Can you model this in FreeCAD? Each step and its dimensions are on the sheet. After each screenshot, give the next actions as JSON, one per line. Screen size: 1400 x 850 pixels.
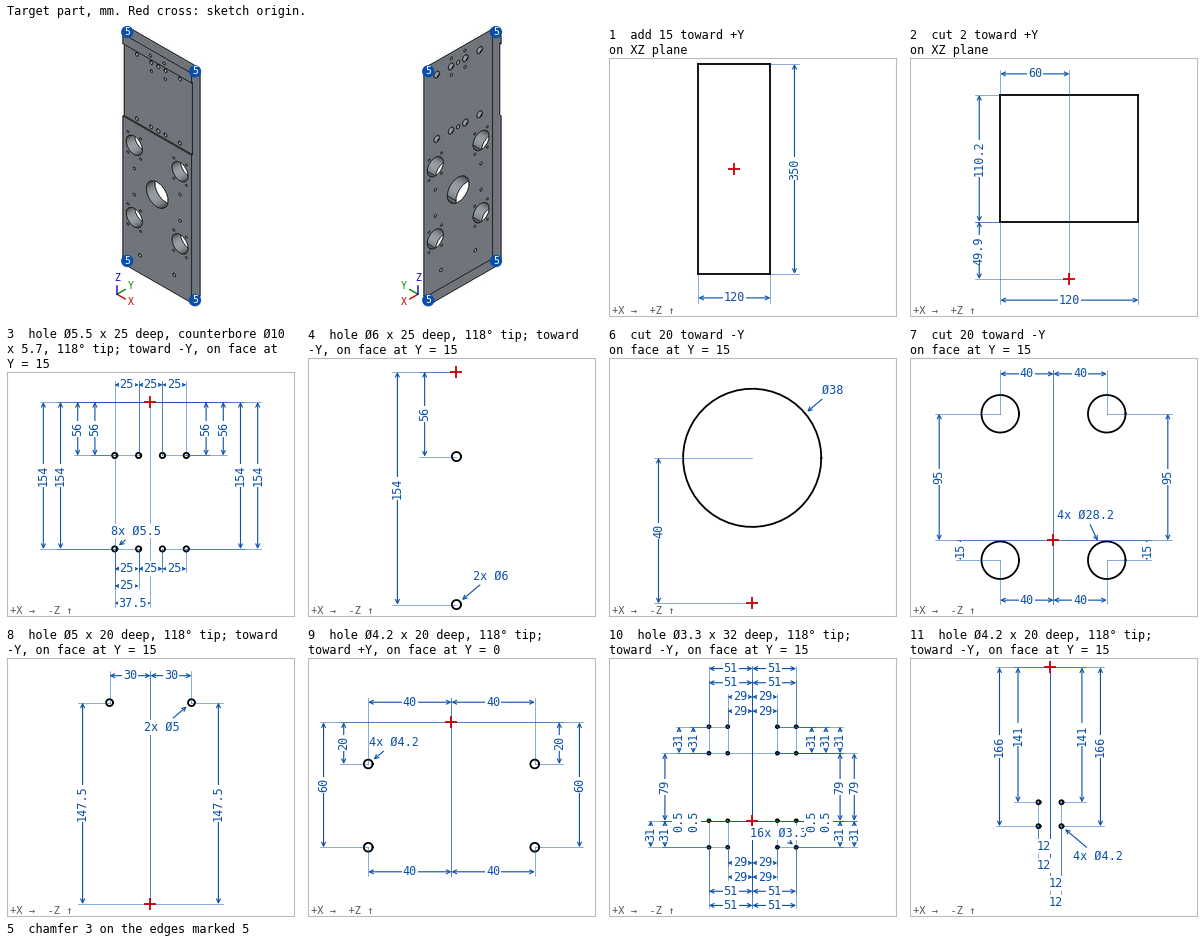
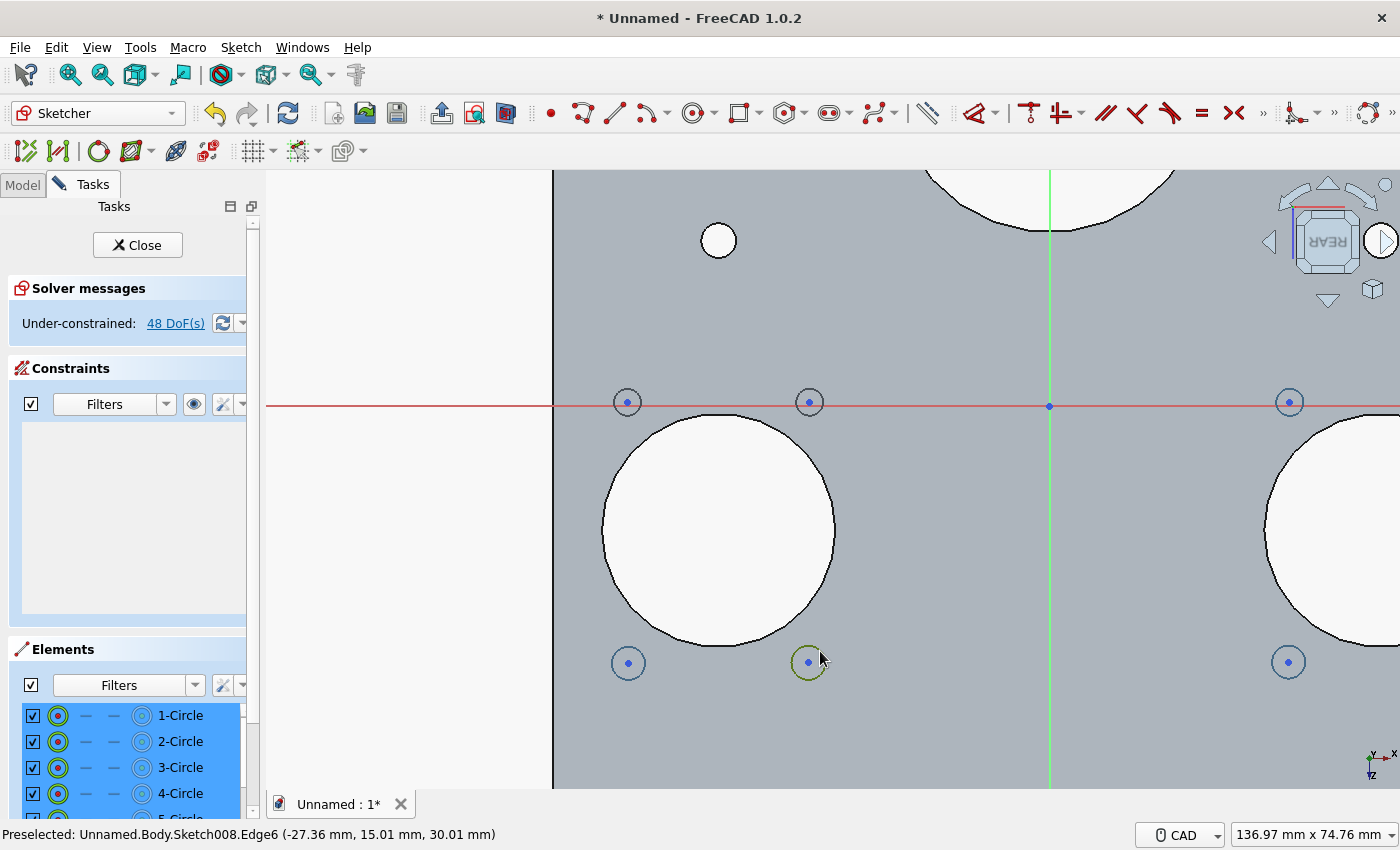
{"action": "left_click", "coordinate": [819, 393]}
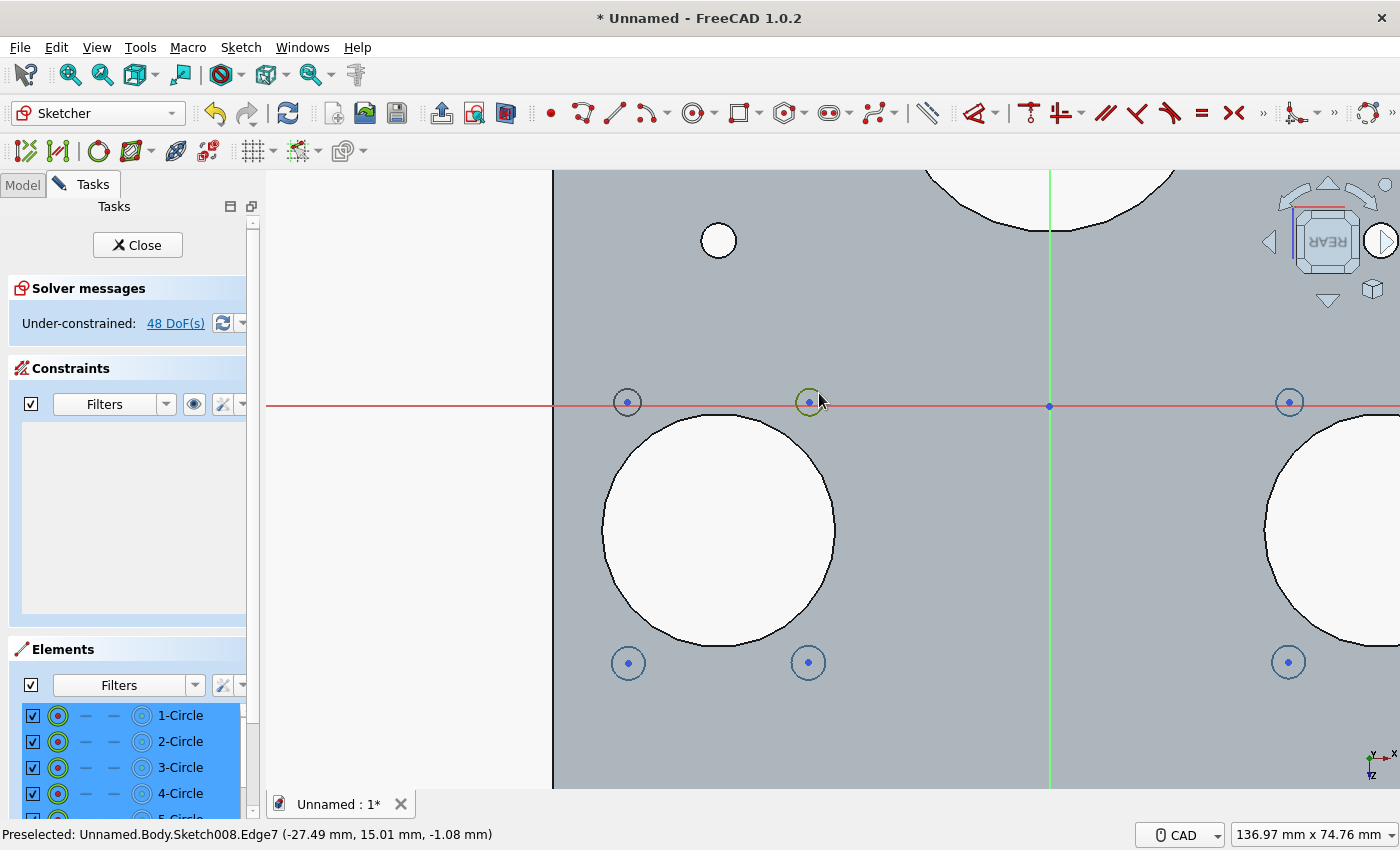
{"action": "left_click", "coordinate": [637, 393]}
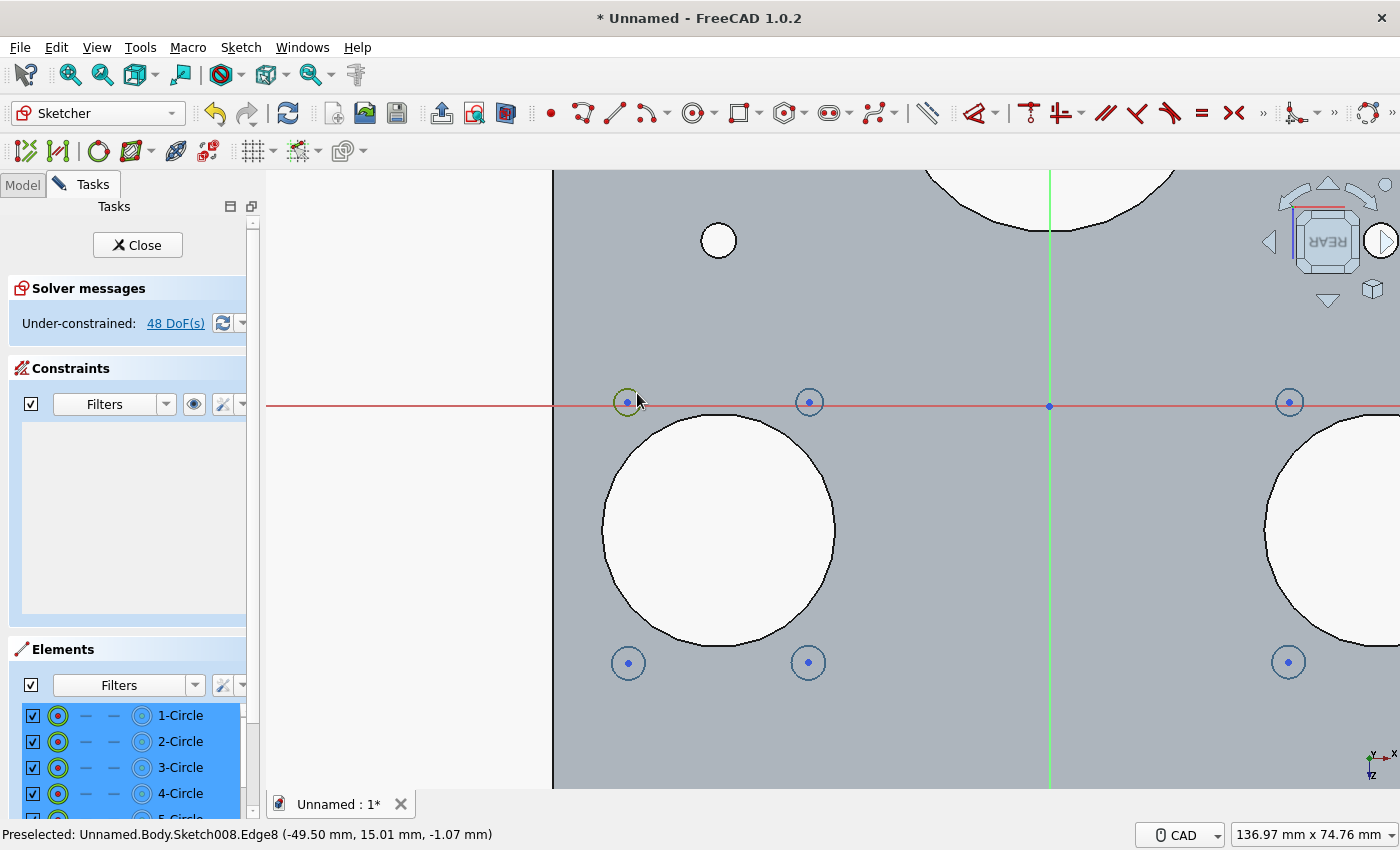
{"action": "scroll", "coordinate": [642, 654], "scroll_direction": "down", "scroll_amount": 6}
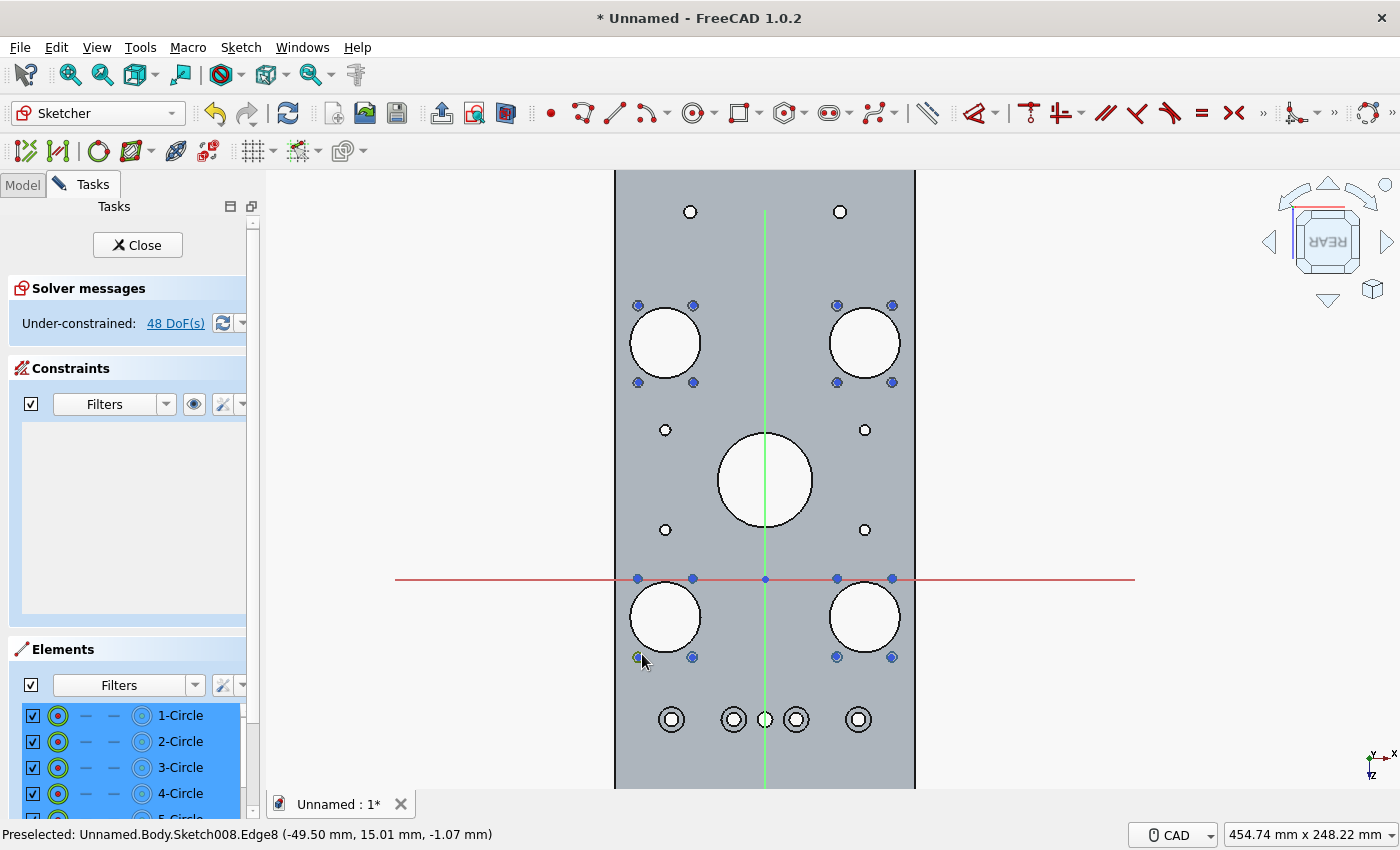
{"action": "scroll", "coordinate": [895, 379], "scroll_direction": "up", "scroll_amount": 6}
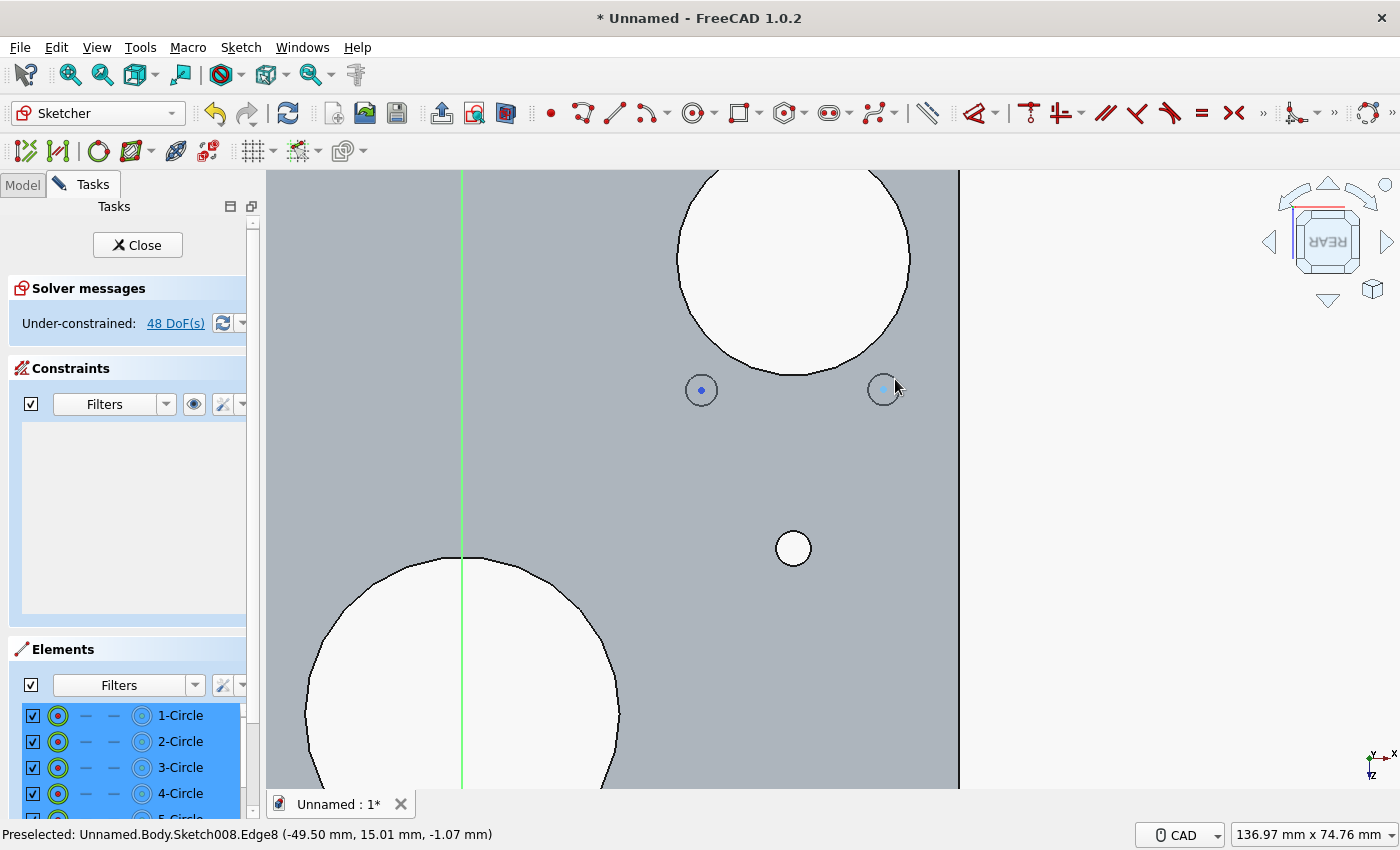
{"action": "left_click", "coordinate": [895, 379]}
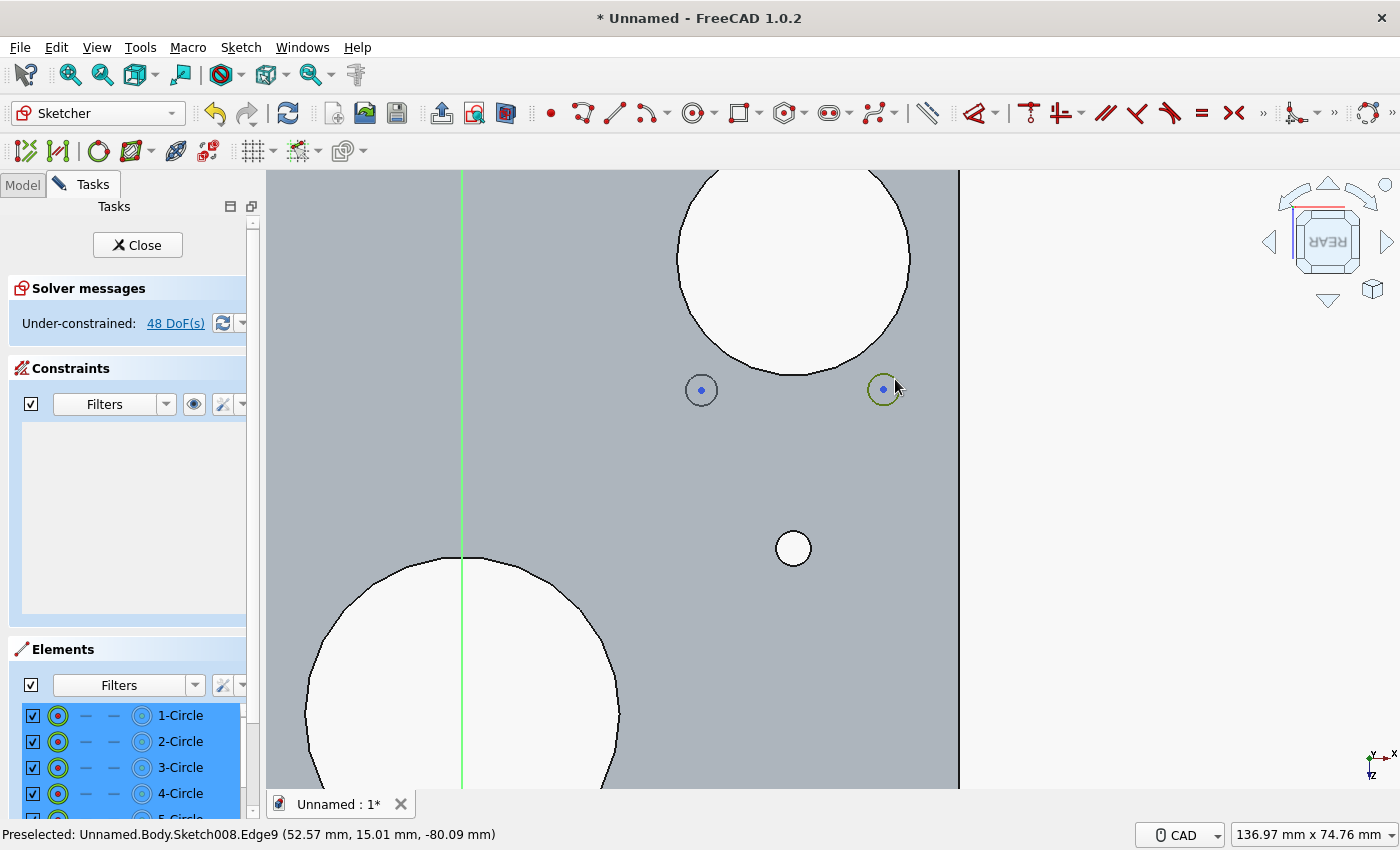
{"action": "left_click", "coordinate": [713, 379]}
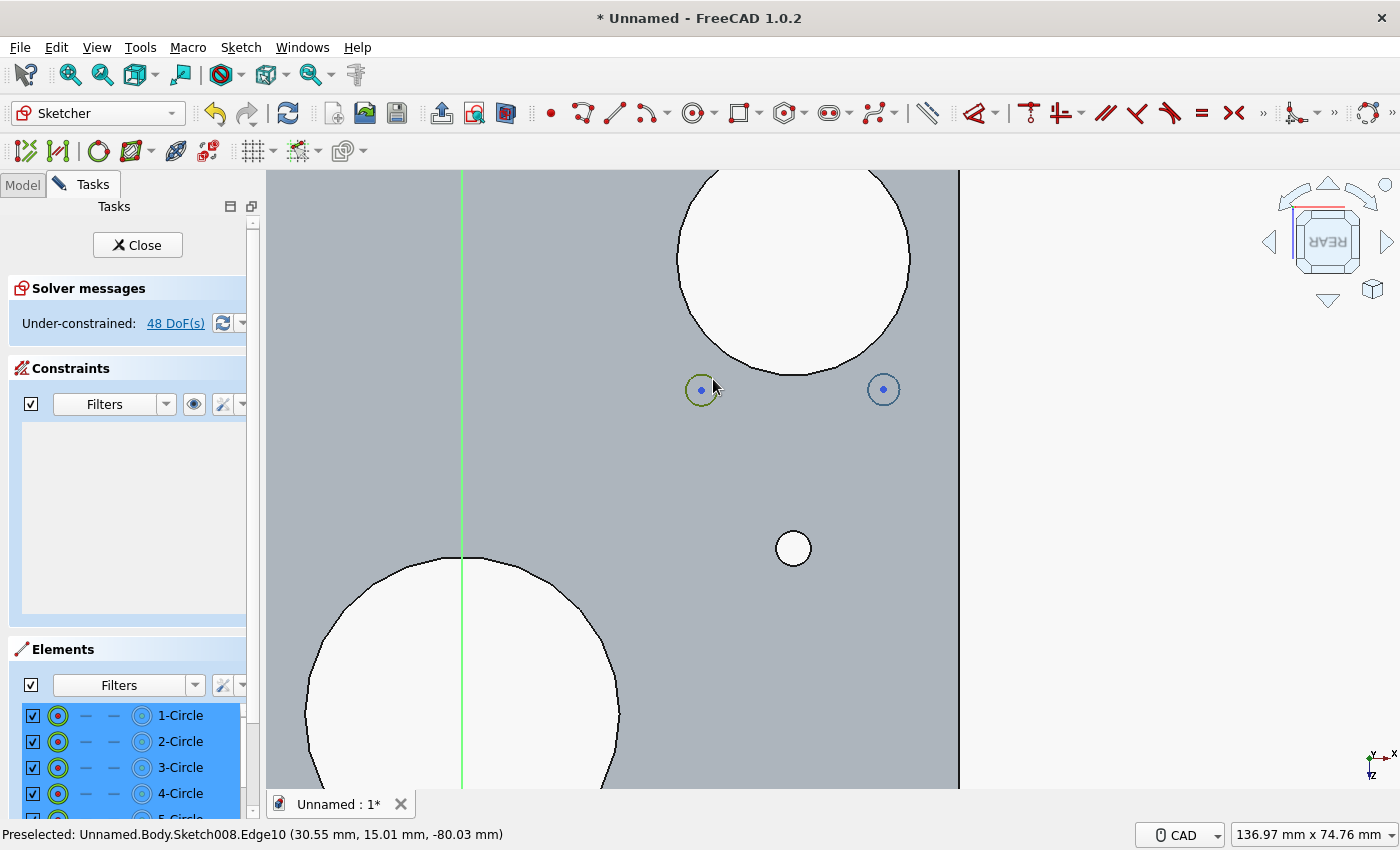
{"action": "scroll", "coordinate": [895, 378], "scroll_direction": "down", "scroll_amount": 6}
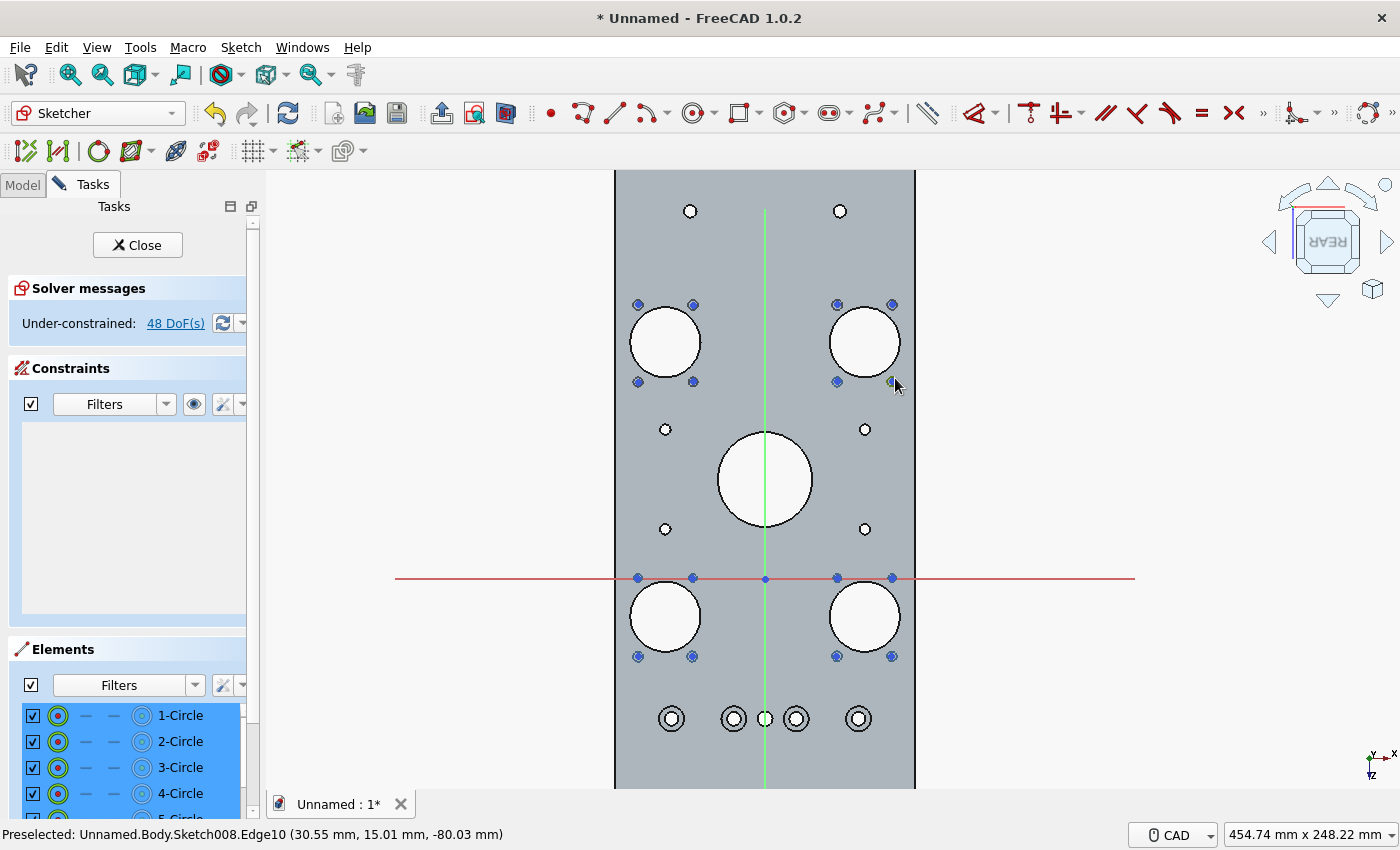
{"action": "scroll", "coordinate": [896, 301], "scroll_direction": "up", "scroll_amount": 6}